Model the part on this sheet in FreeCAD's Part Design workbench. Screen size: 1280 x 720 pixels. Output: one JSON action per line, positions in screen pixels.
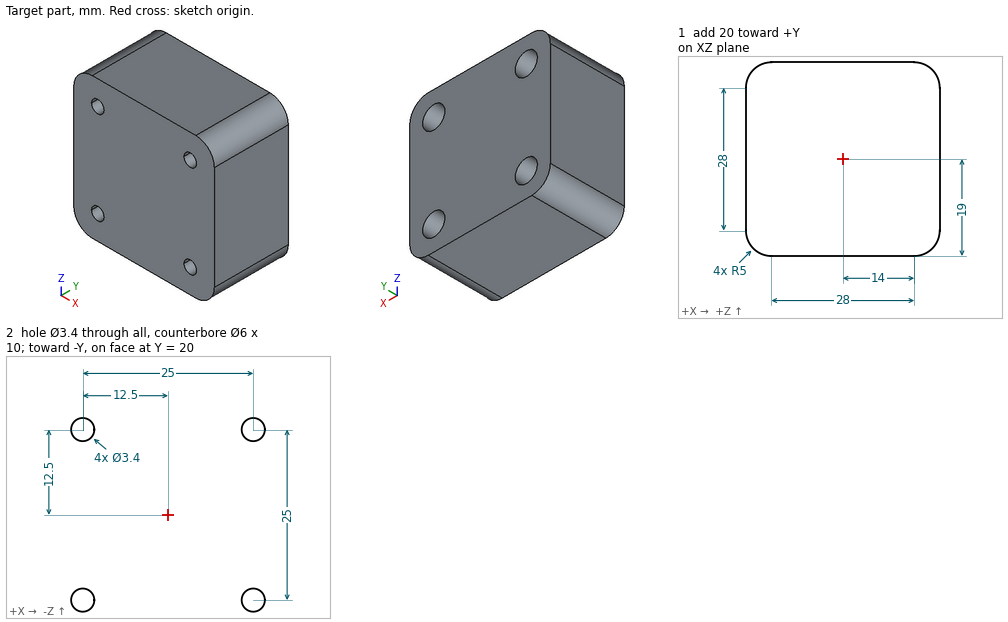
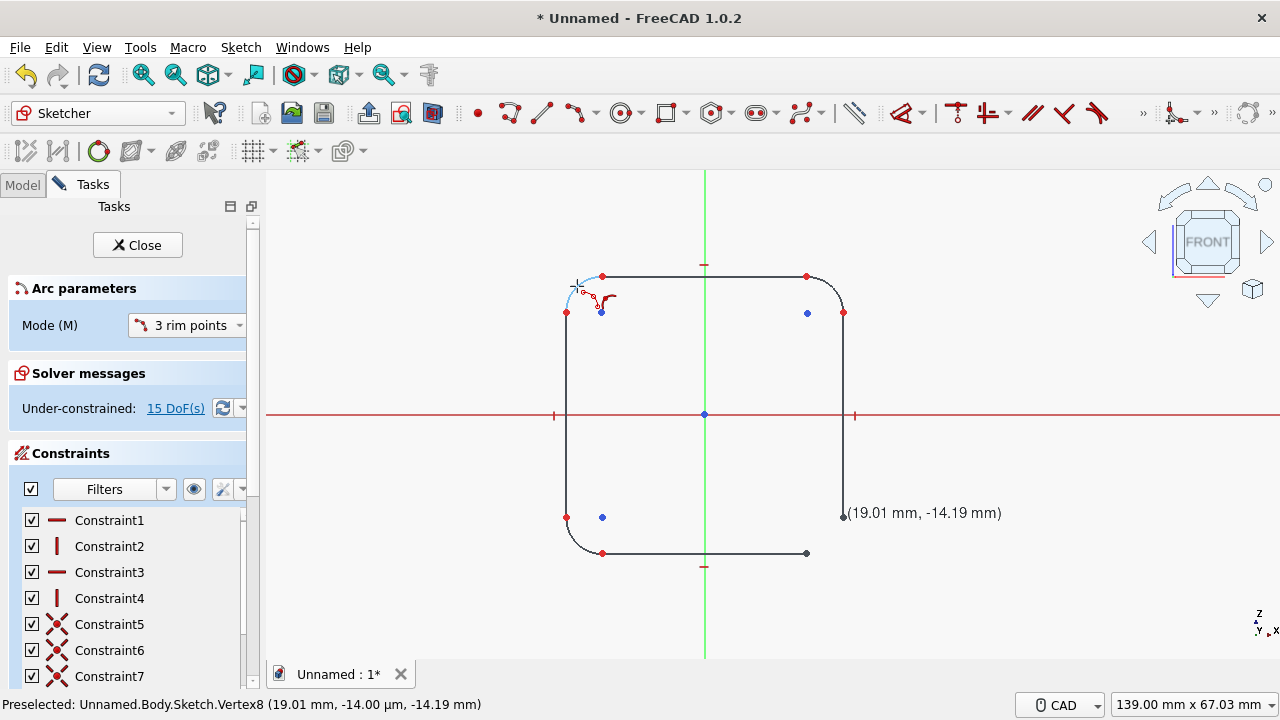
{"action": "left_click", "coordinate": [806, 554]}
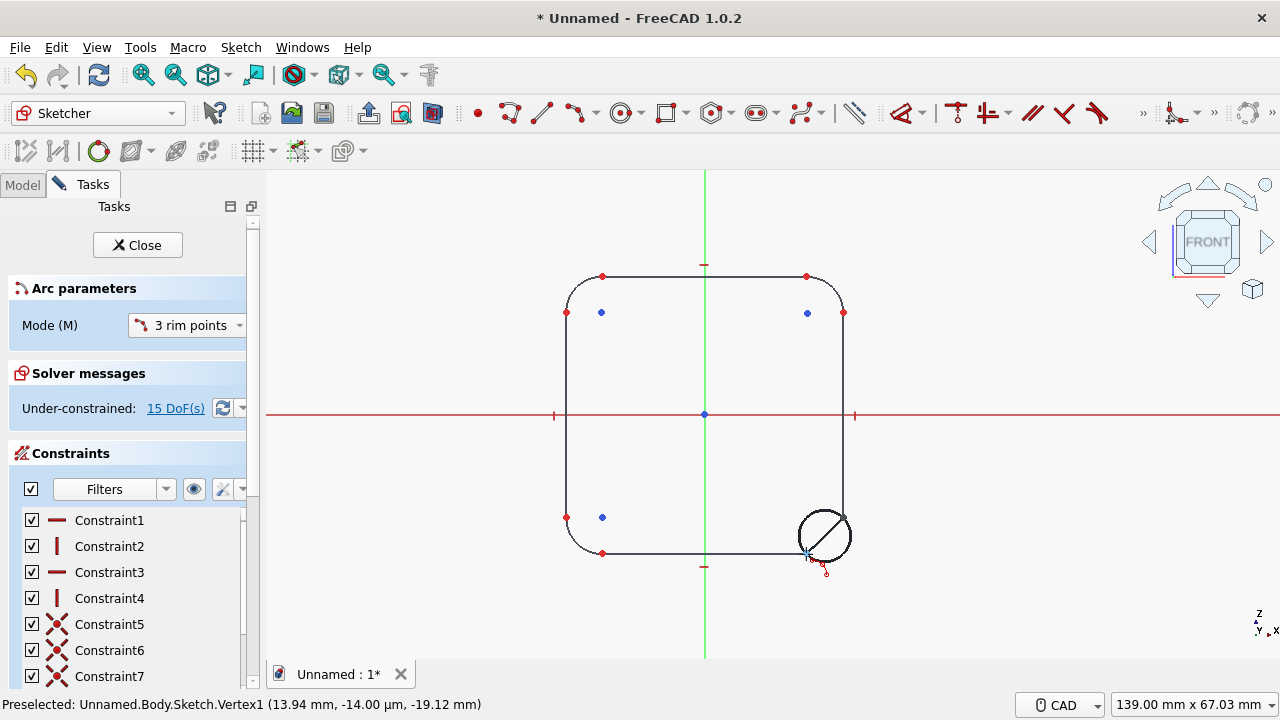
{"action": "scroll", "coordinate": [833, 542], "scroll_direction": "up", "scroll_amount": 2}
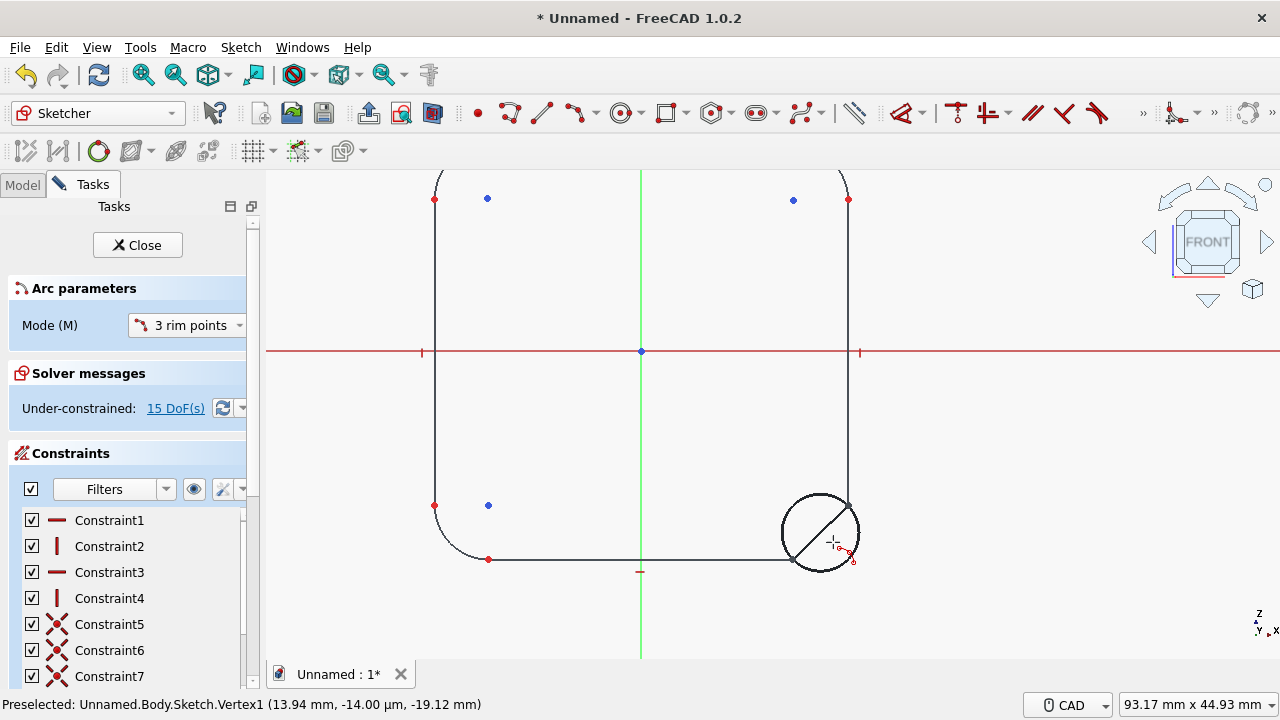
{"action": "left_click", "coordinate": [832, 542]}
{"action": "key", "text": "Escape"}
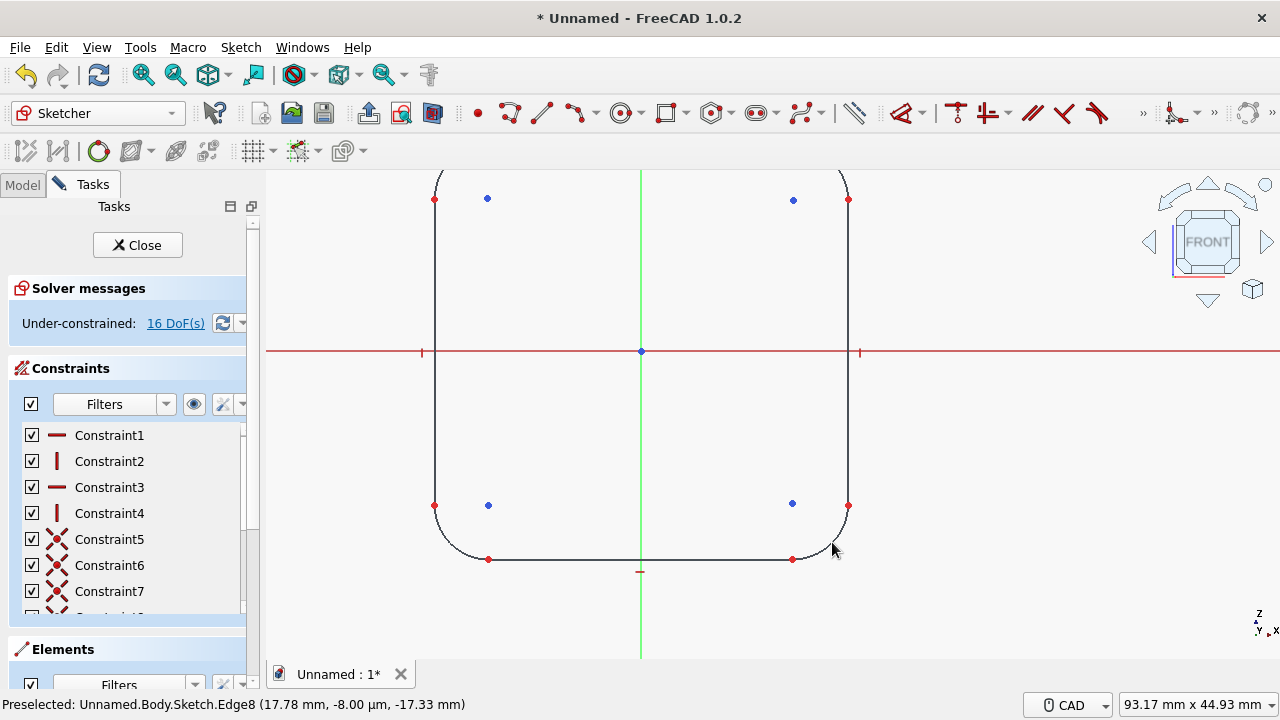
{"action": "left_click", "coordinate": [702, 560]}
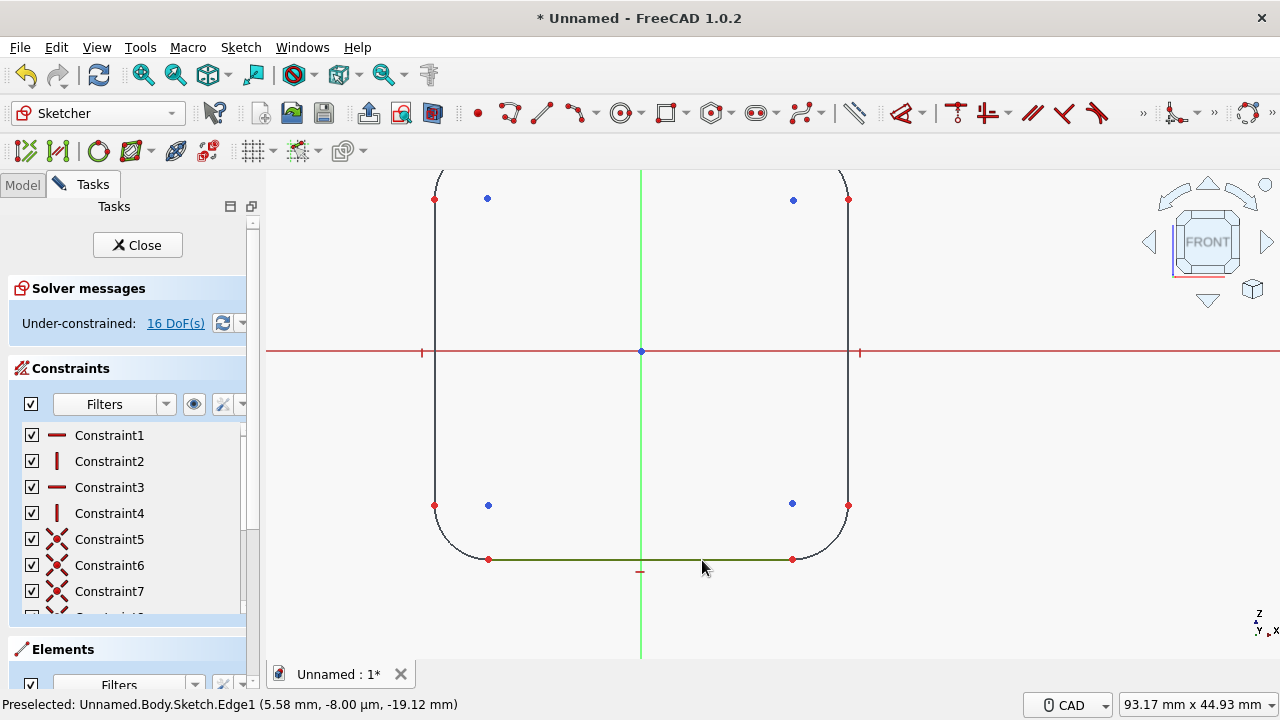
{"action": "left_click", "coordinate": [441, 530]}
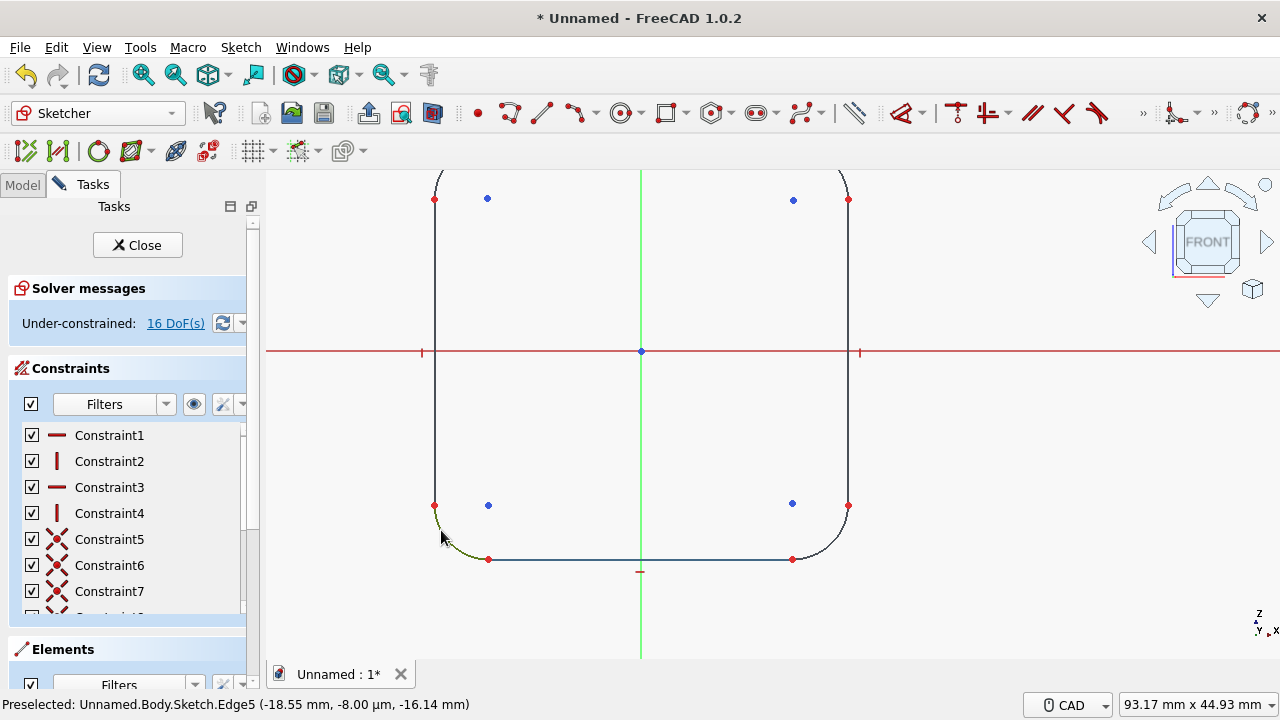
{"action": "left_click", "coordinate": [1098, 114]}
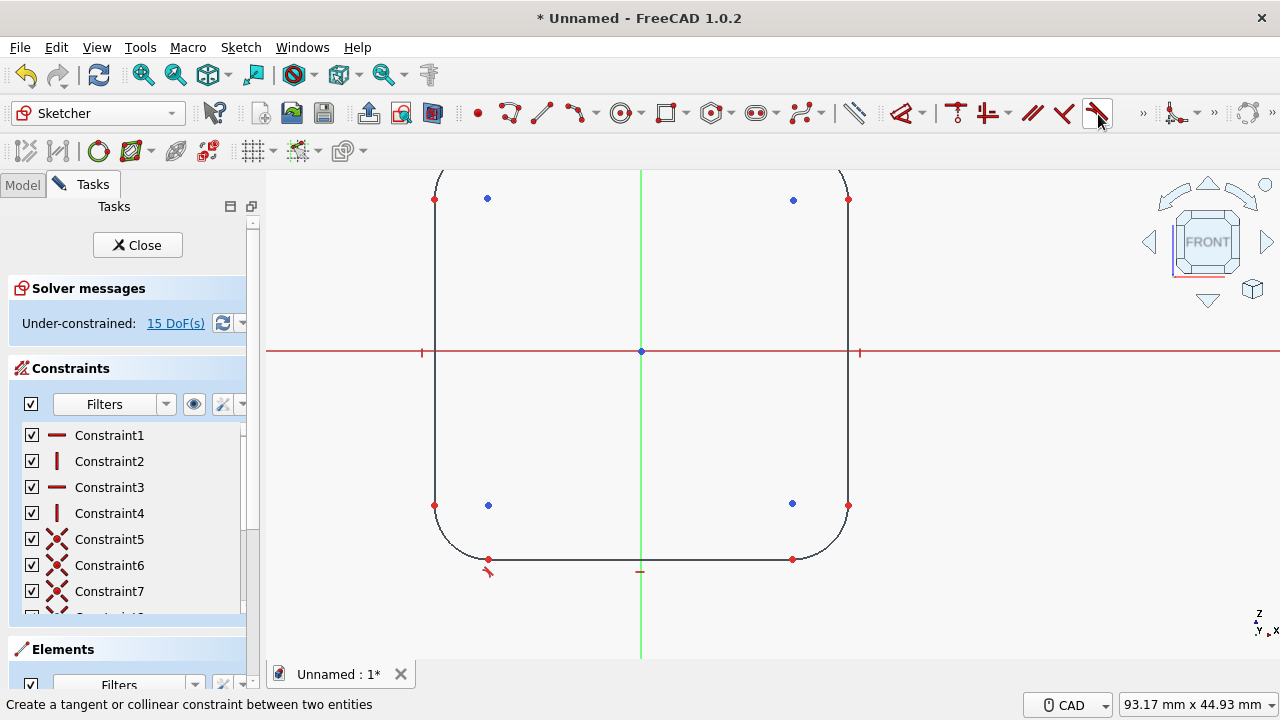
{"action": "left_click", "coordinate": [702, 560]}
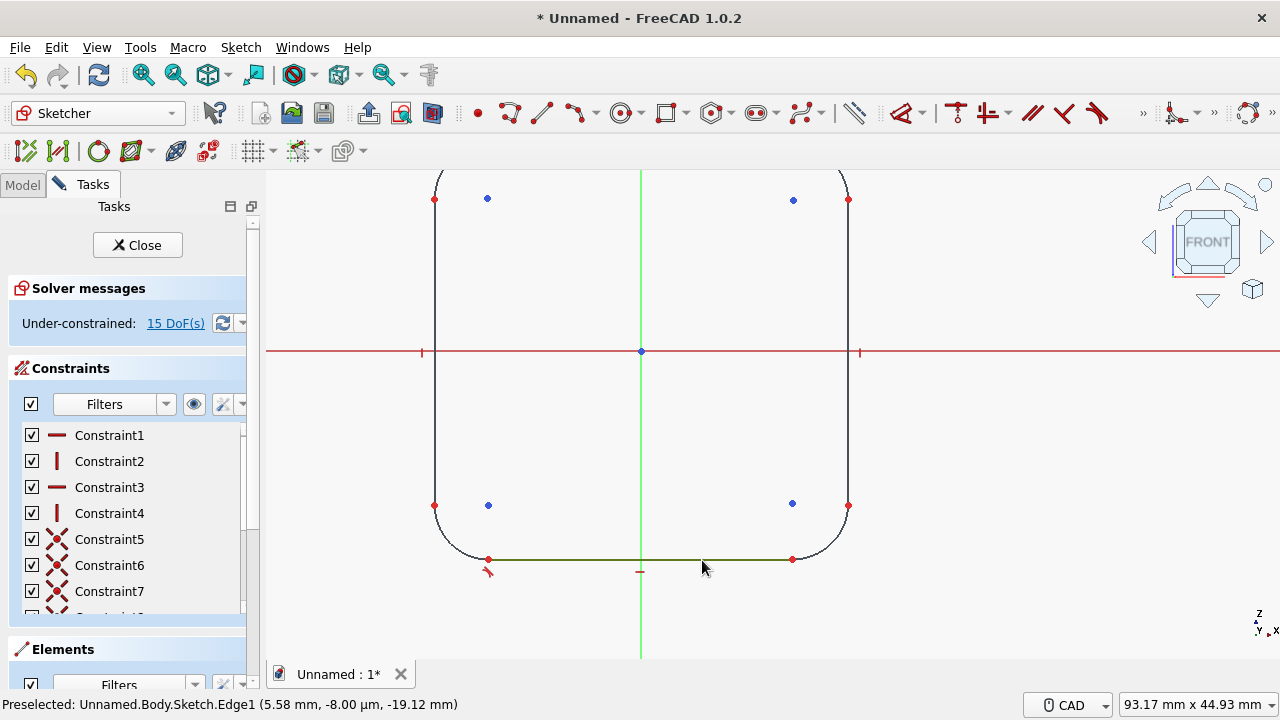
{"action": "left_click", "coordinate": [817, 554]}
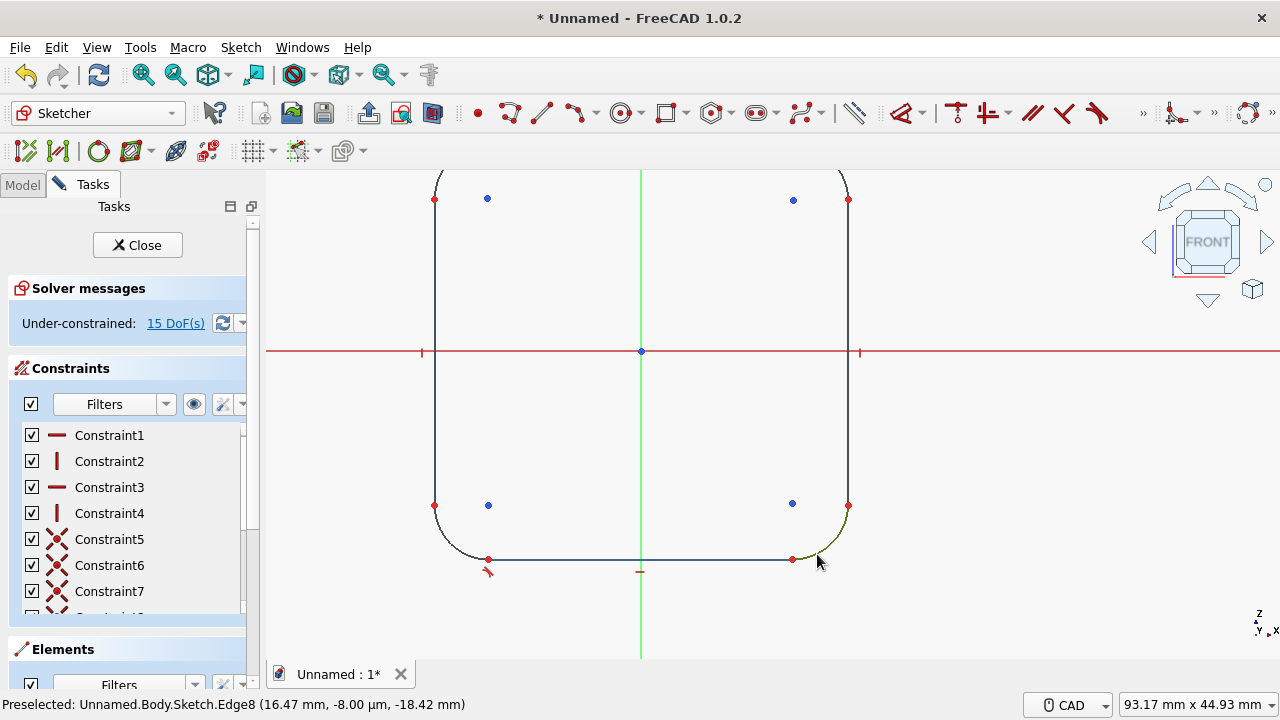
{"action": "left_click", "coordinate": [1098, 114]}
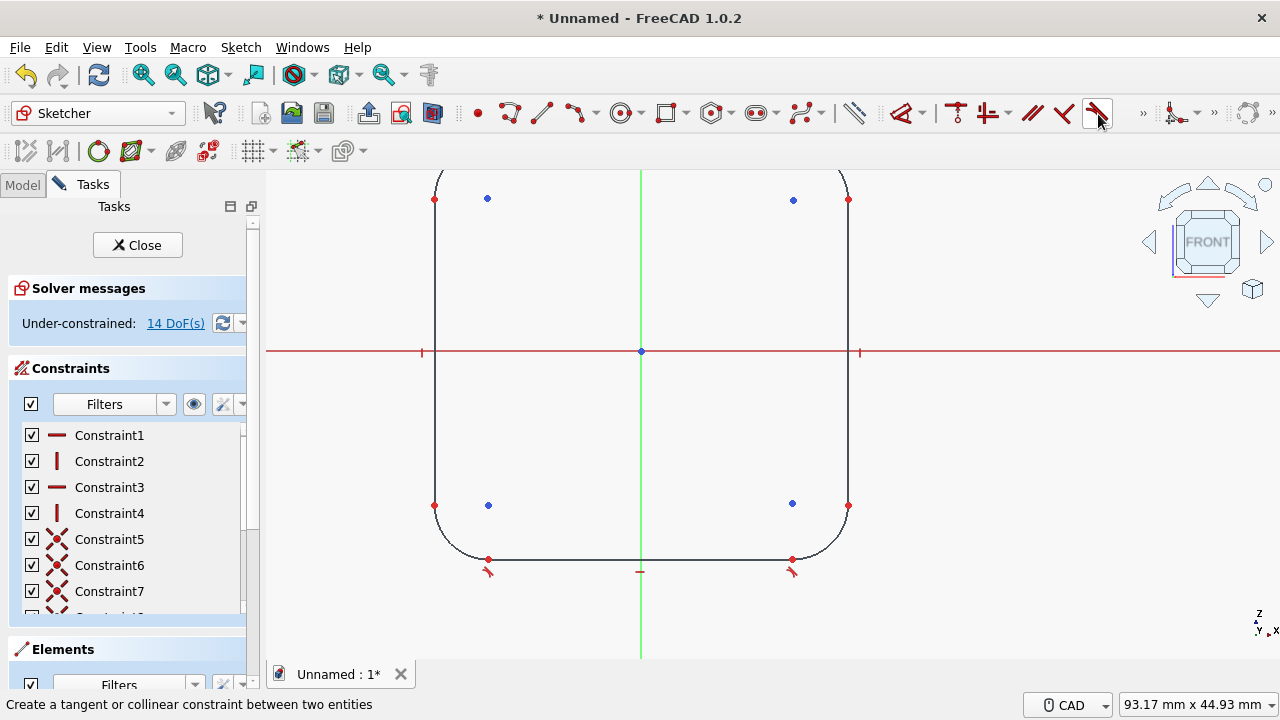
{"action": "left_click", "coordinate": [435, 414]}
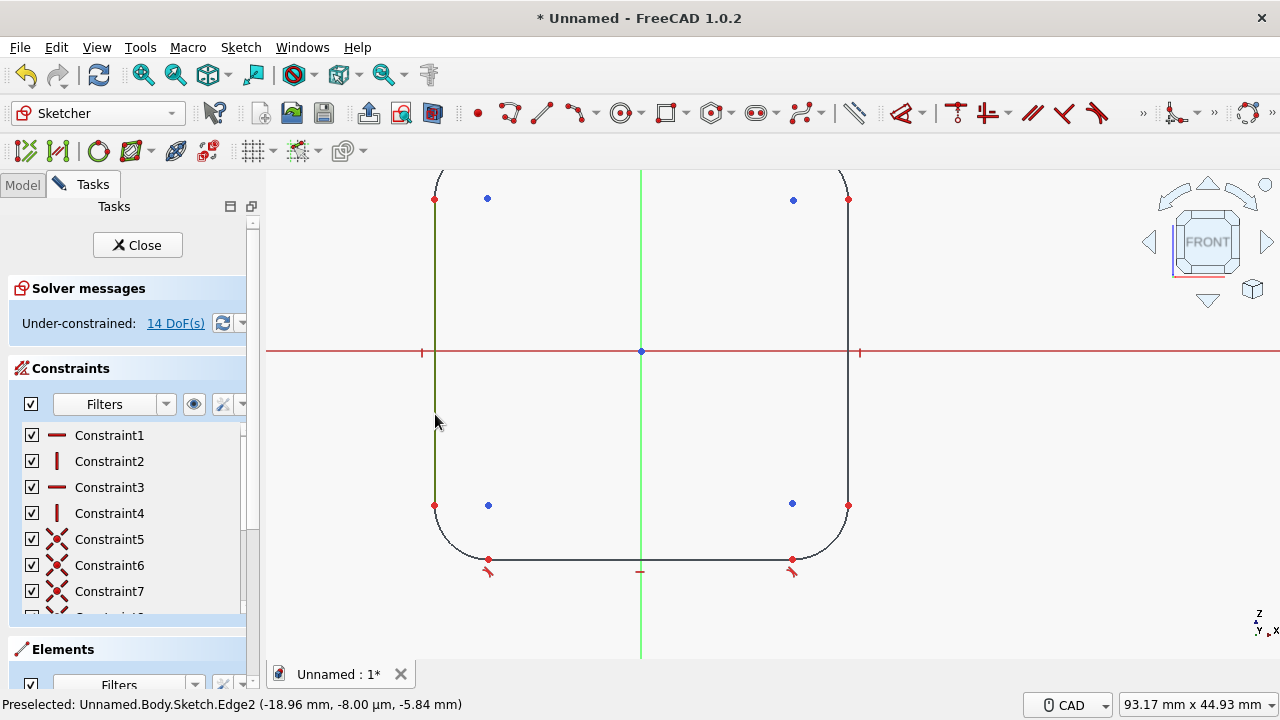
{"action": "left_click", "coordinate": [441, 530]}